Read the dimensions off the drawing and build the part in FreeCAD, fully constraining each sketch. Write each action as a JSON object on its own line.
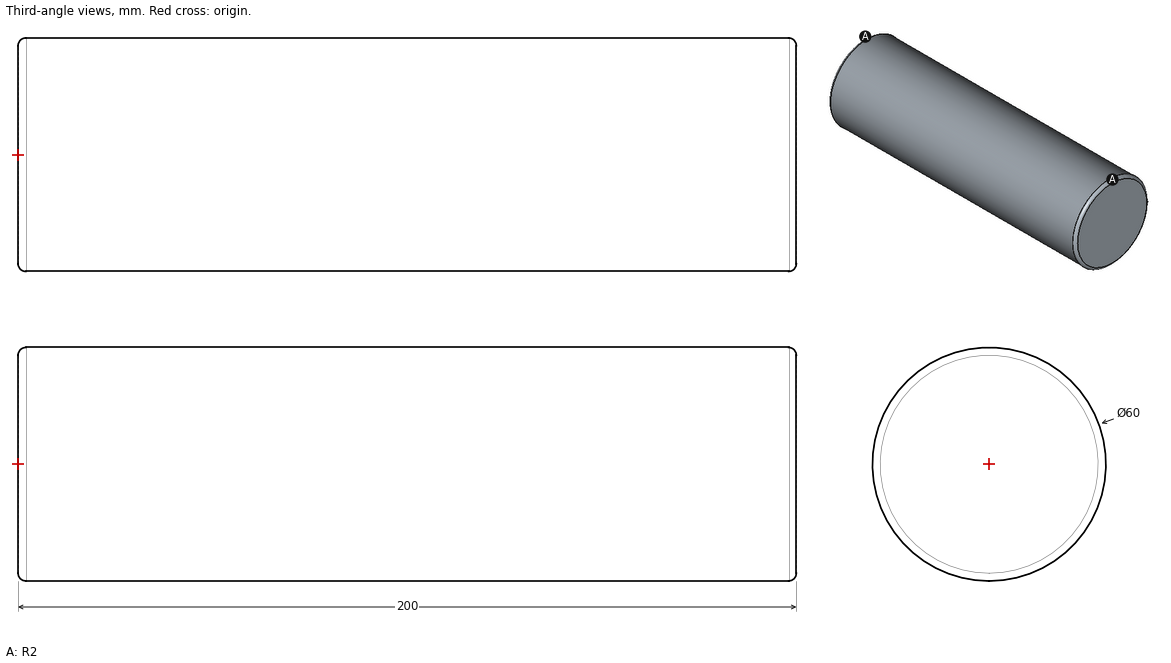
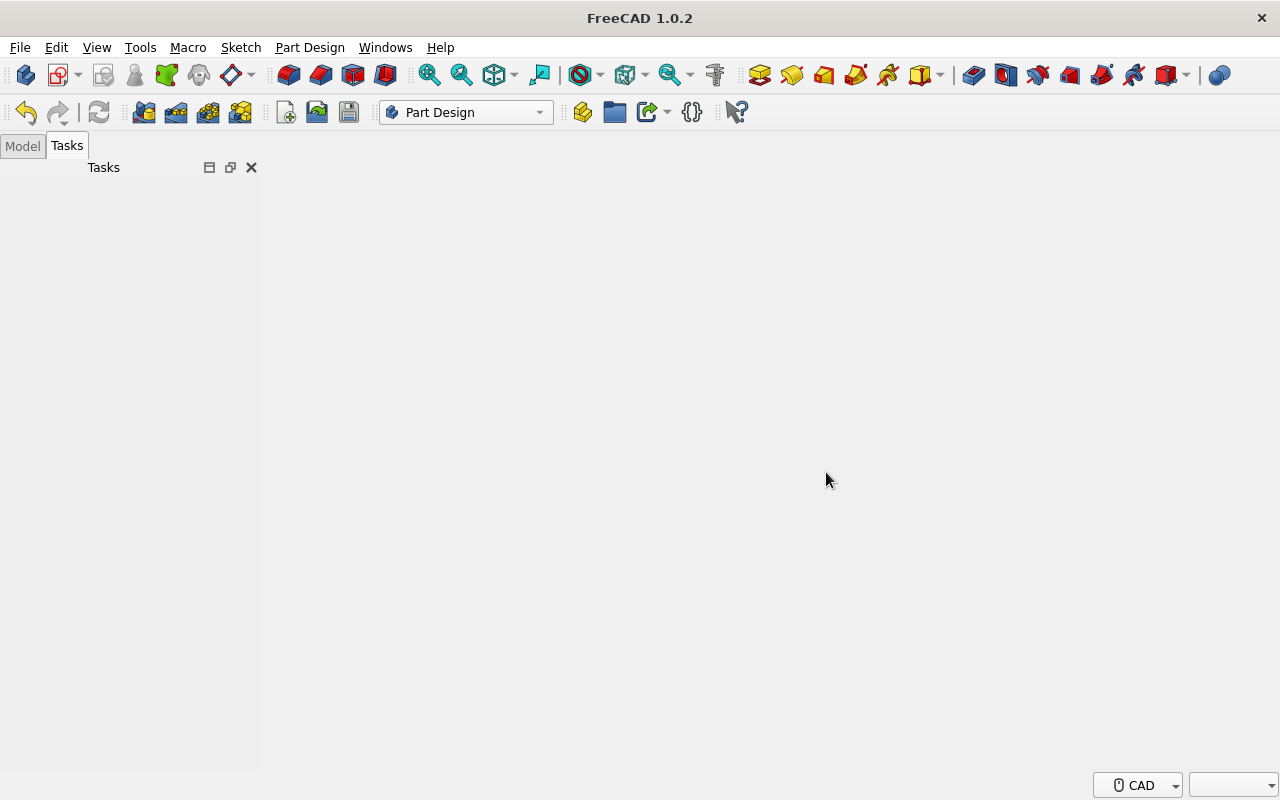
{"action": "left_click", "coordinate": [286, 112]}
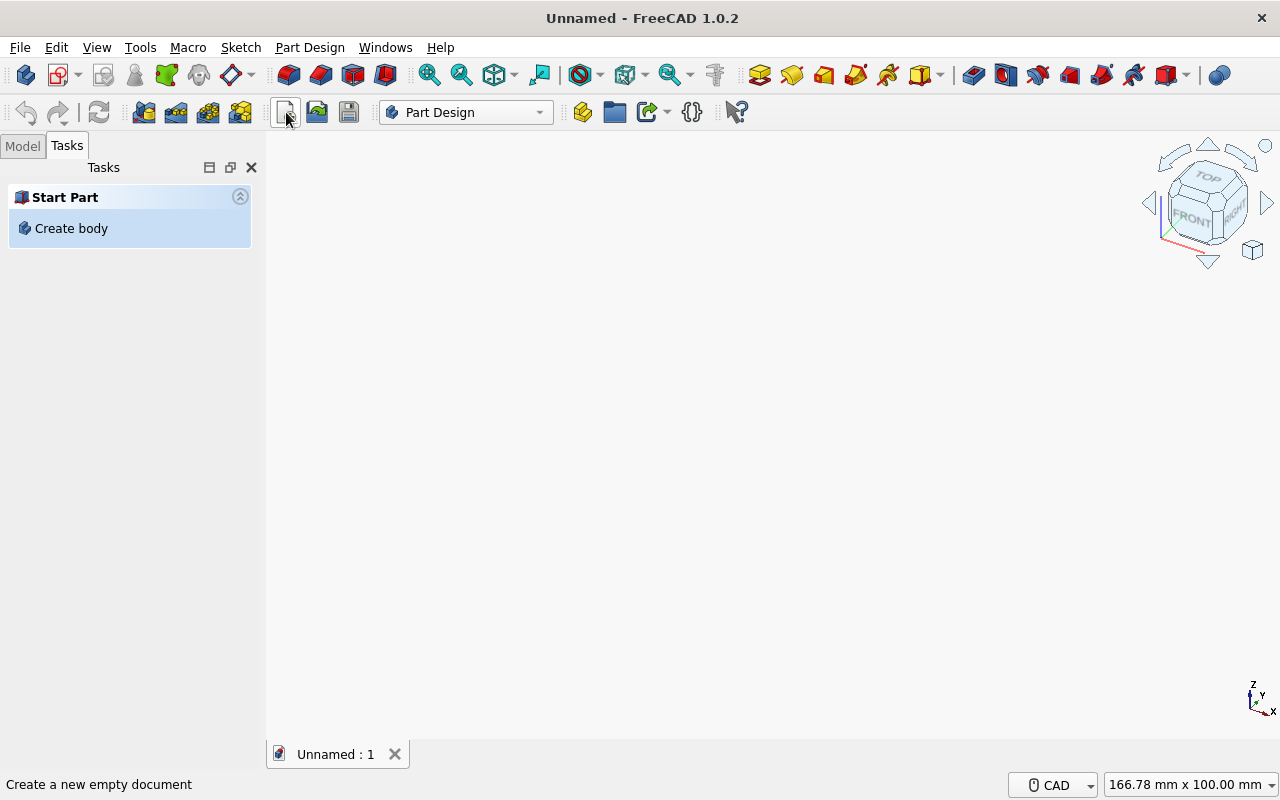
{"action": "left_click", "coordinate": [58, 76]}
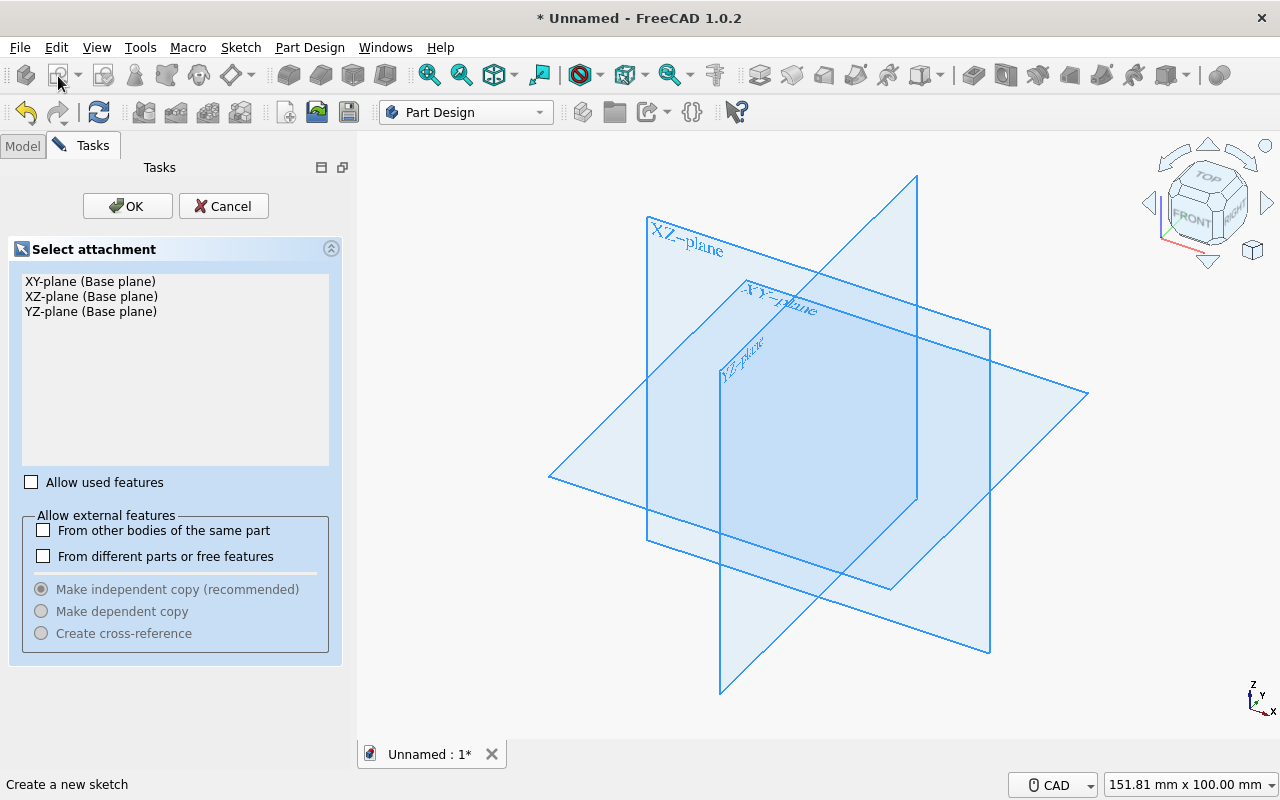
{"action": "left_click", "coordinate": [82, 312]}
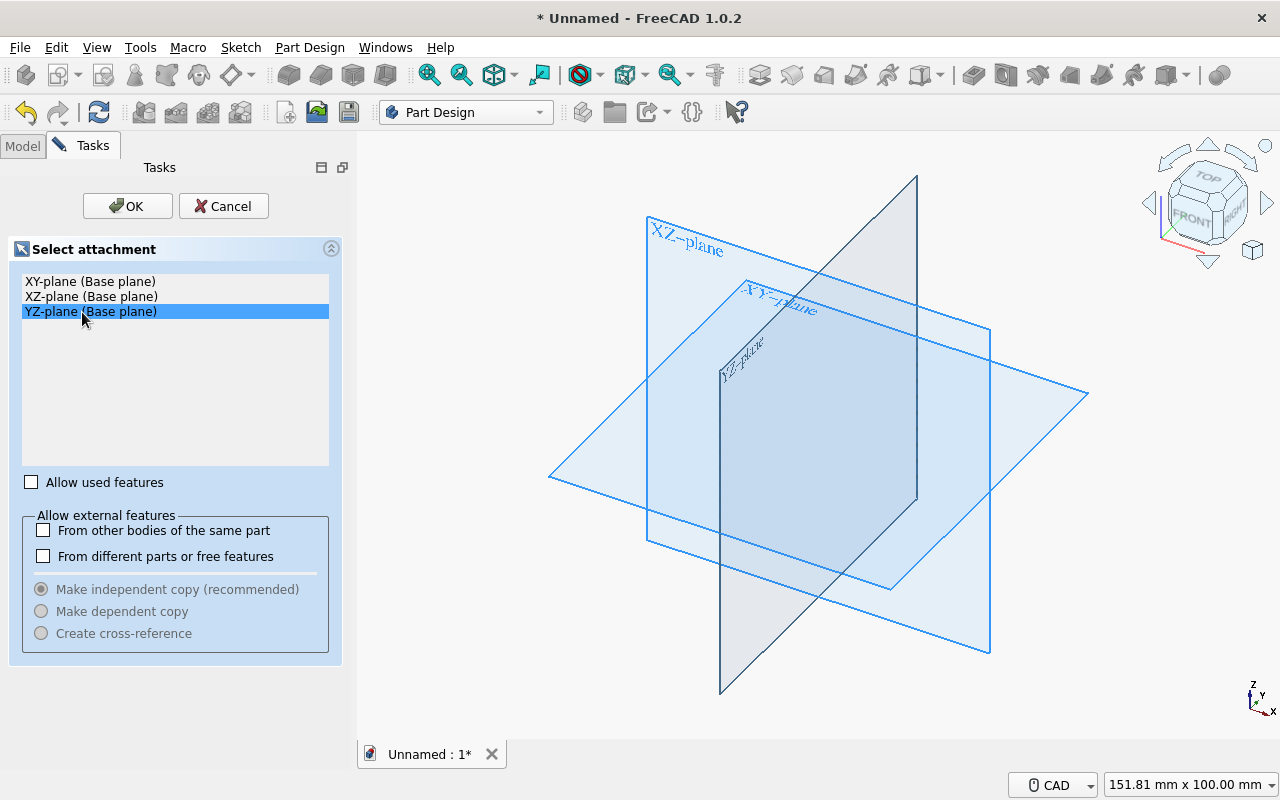
{"action": "left_click", "coordinate": [128, 206]}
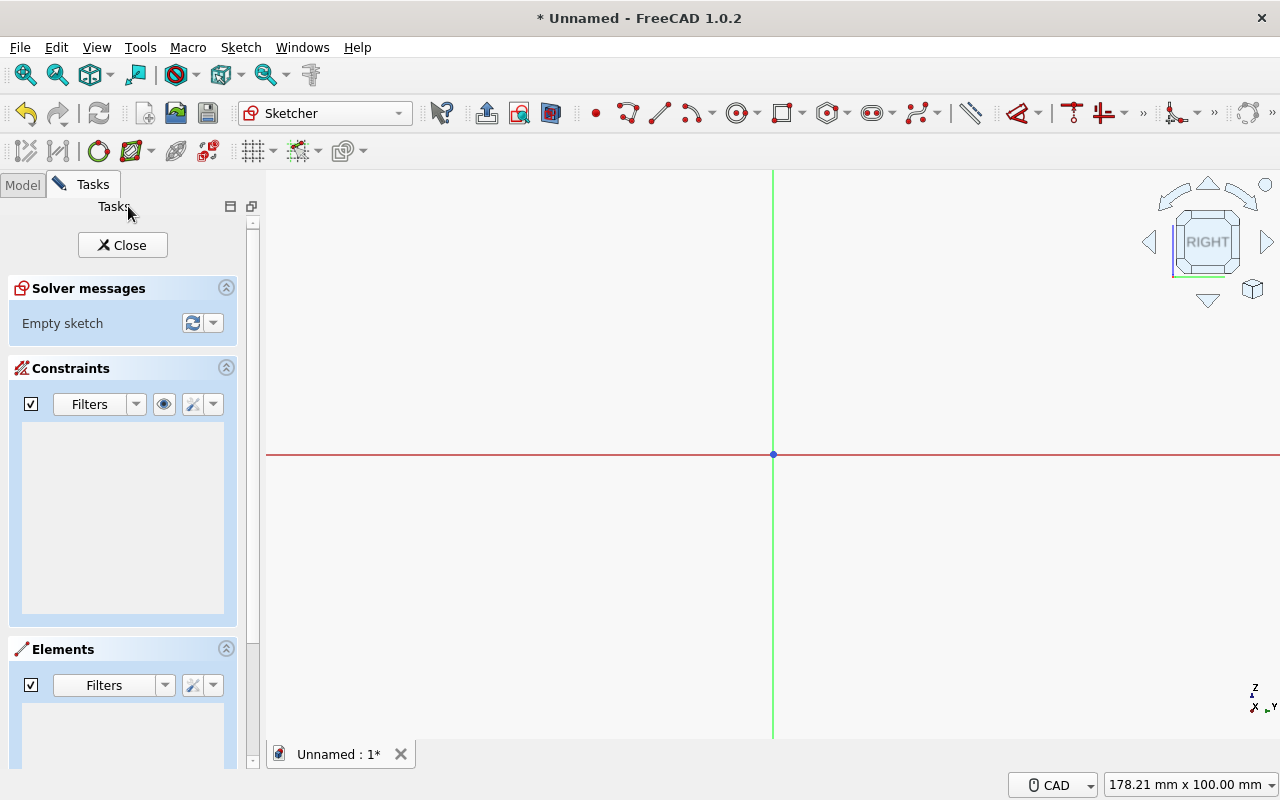
{"action": "left_click", "coordinate": [738, 114]}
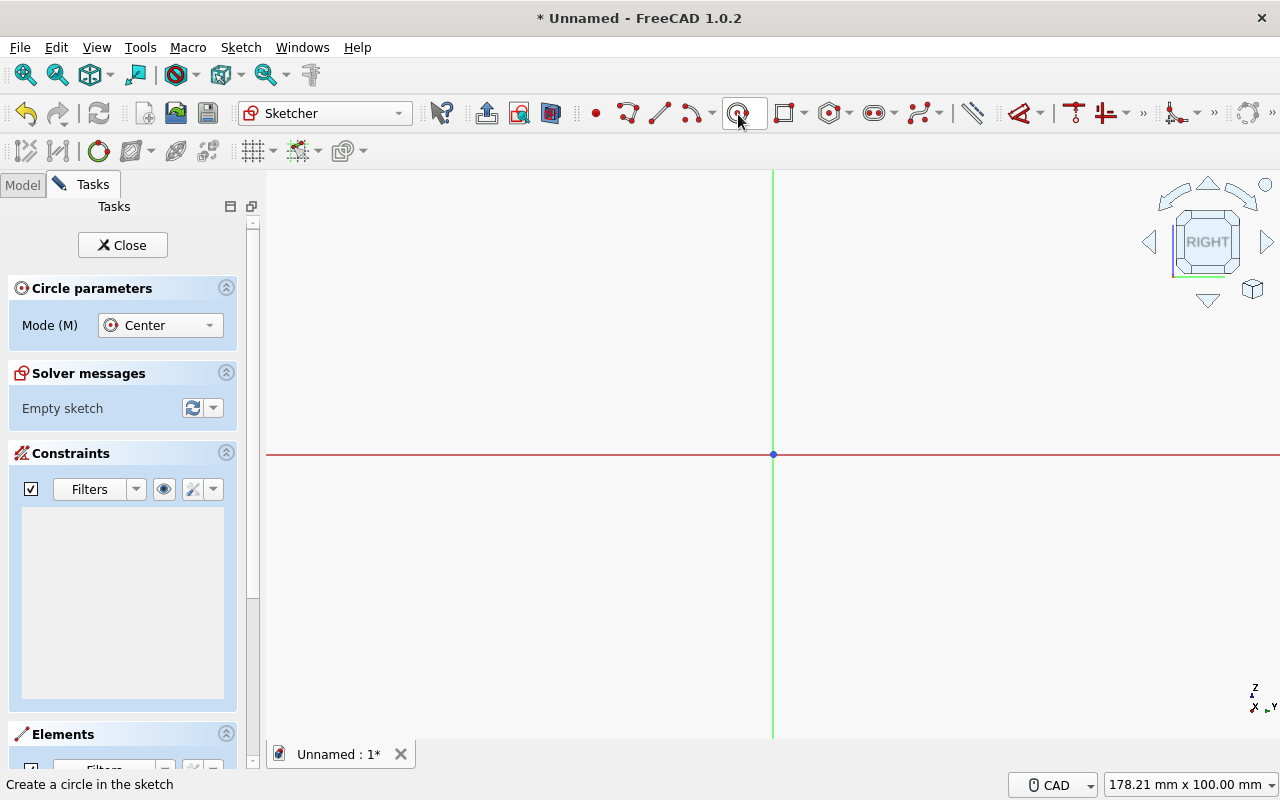
{"action": "left_click", "coordinate": [773, 454]}
{"action": "mouse_move", "coordinate": [894, 334]}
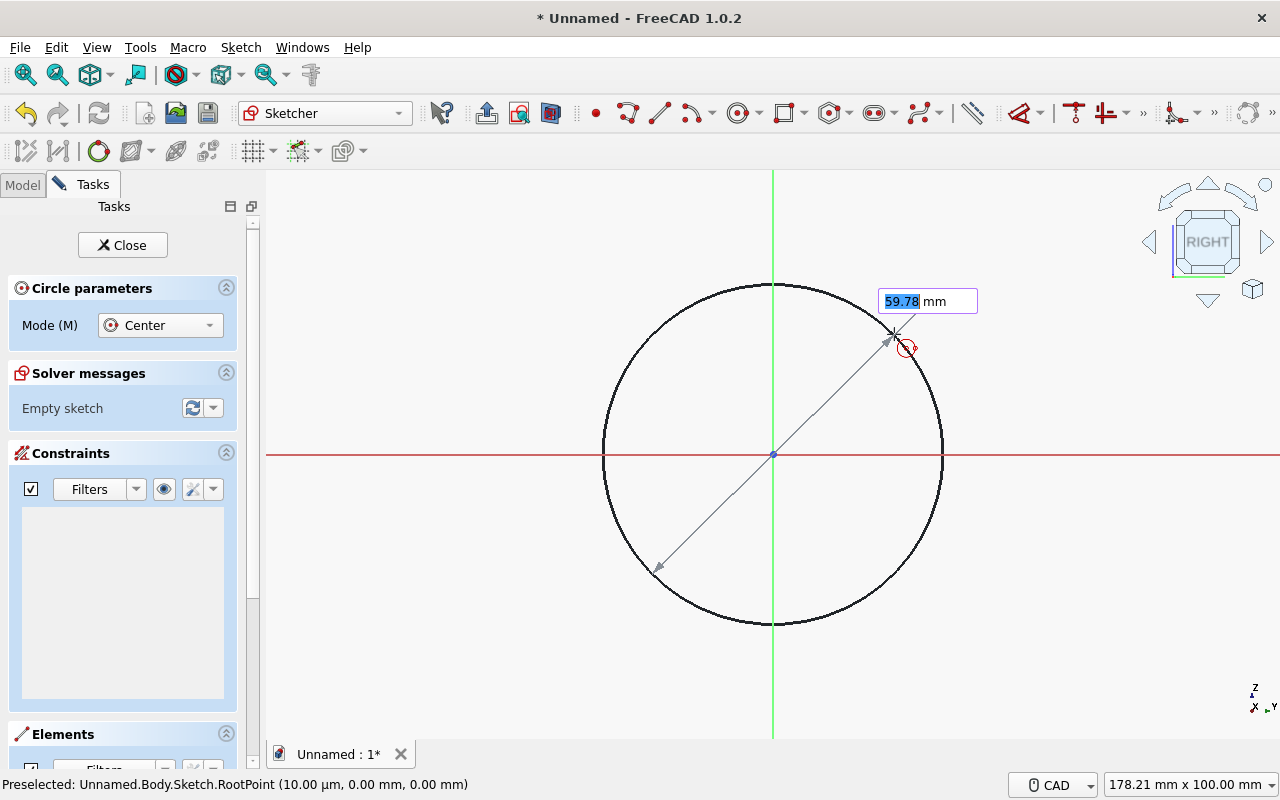
{"action": "type", "text": "60"}
{"action": "key", "text": "Return"}
{"action": "key", "text": "Escape"}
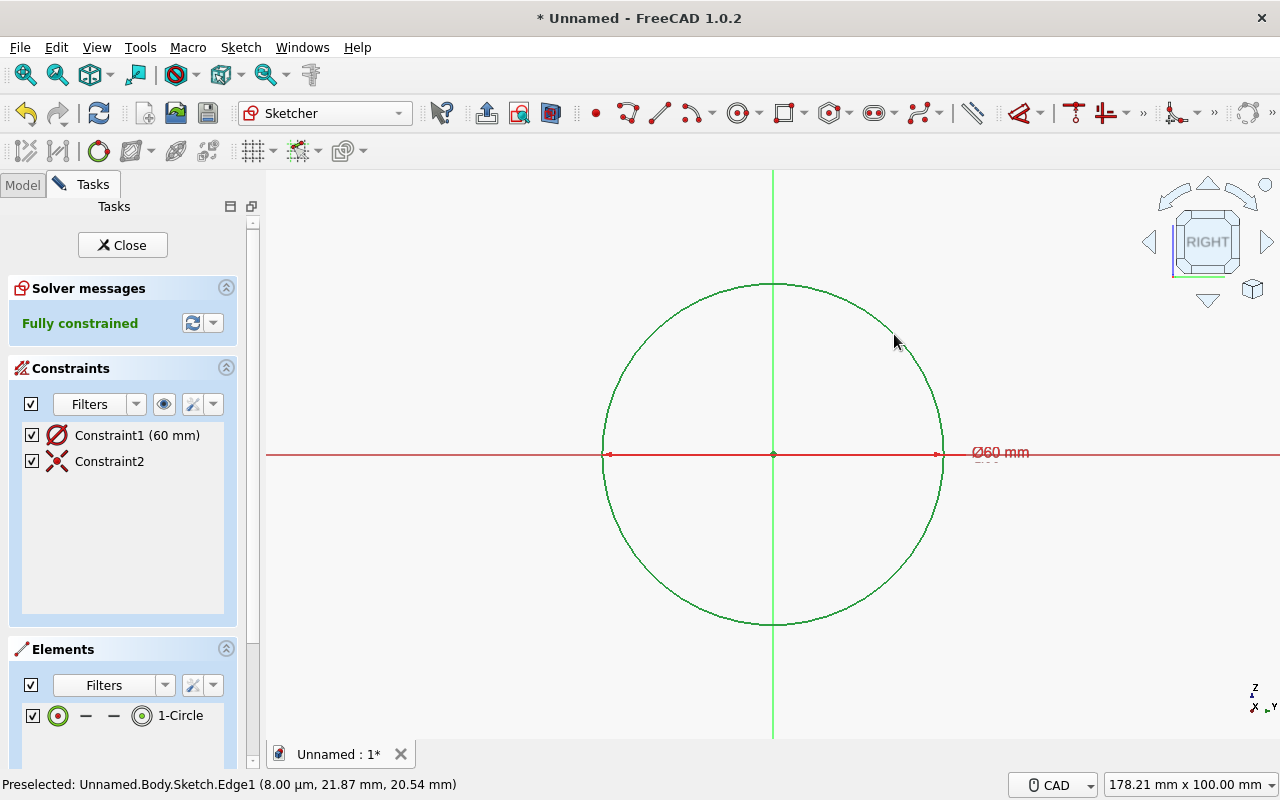
{"action": "left_click", "coordinate": [123, 245]}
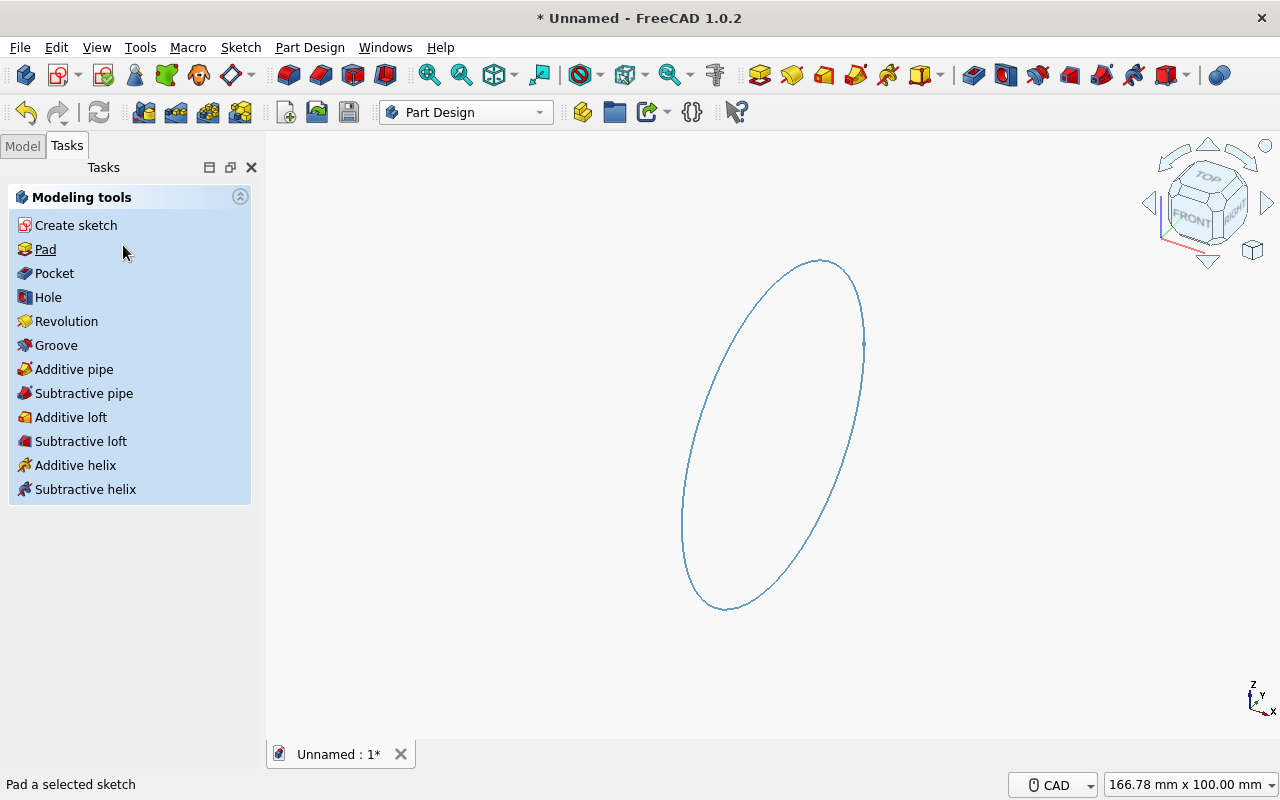
{"action": "left_click", "coordinate": [760, 76]}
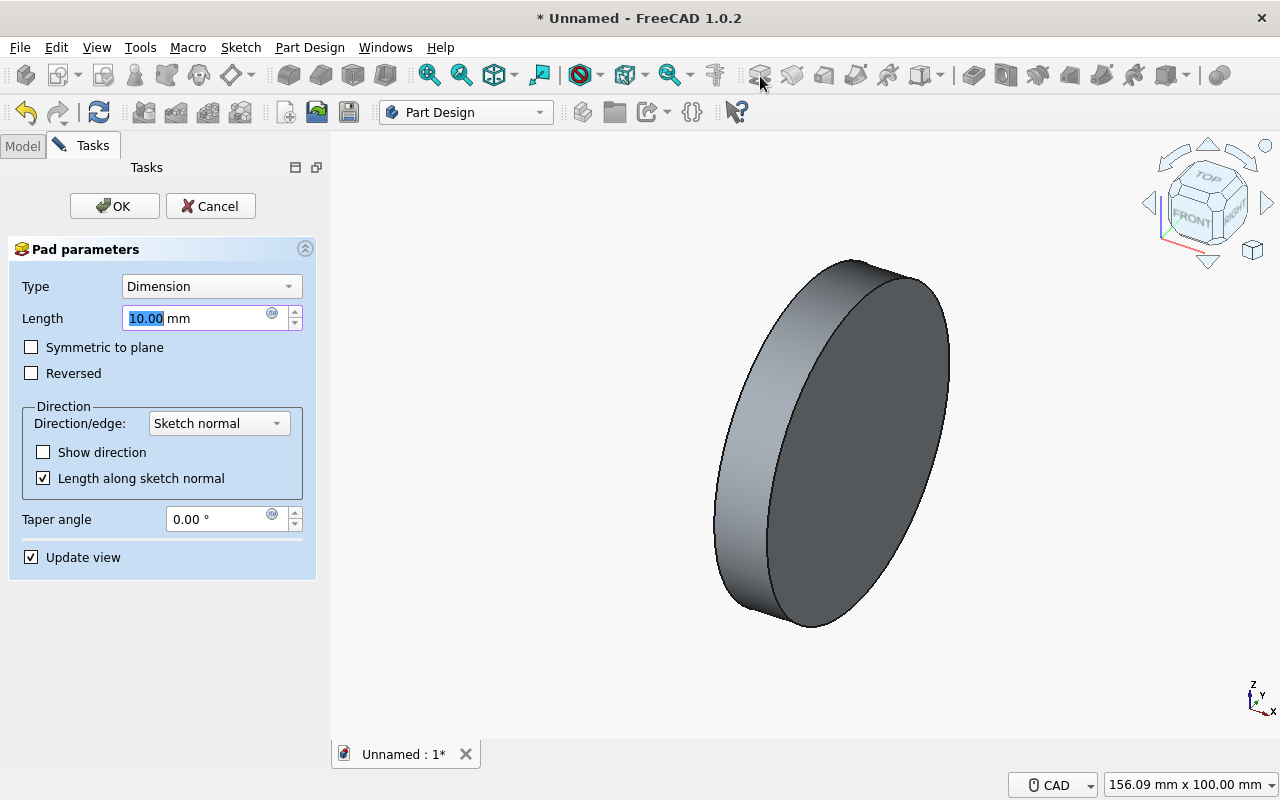
{"action": "type", "text": "200"}
{"action": "key", "text": "Tab"}